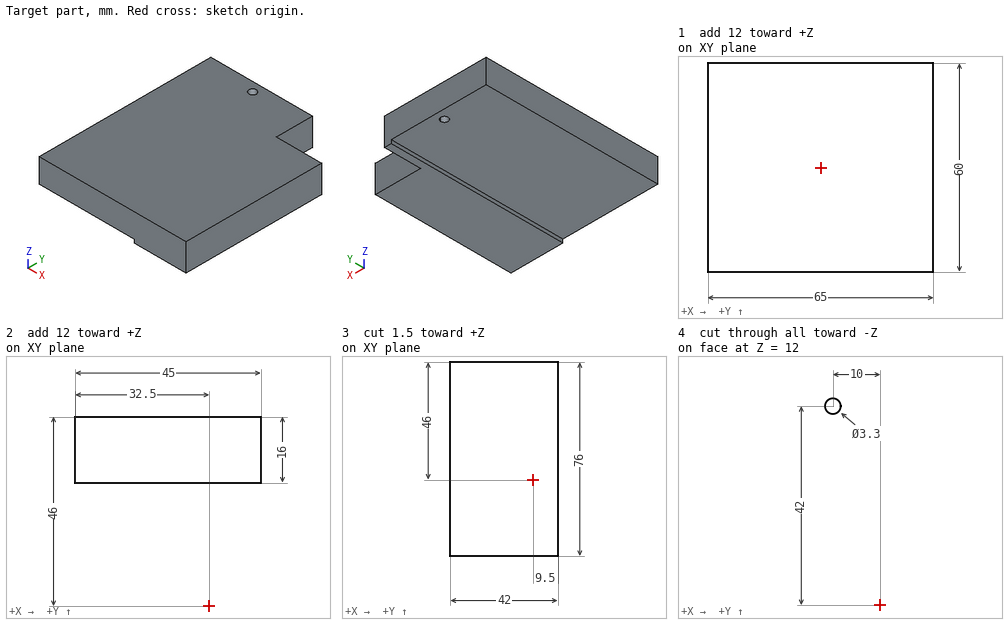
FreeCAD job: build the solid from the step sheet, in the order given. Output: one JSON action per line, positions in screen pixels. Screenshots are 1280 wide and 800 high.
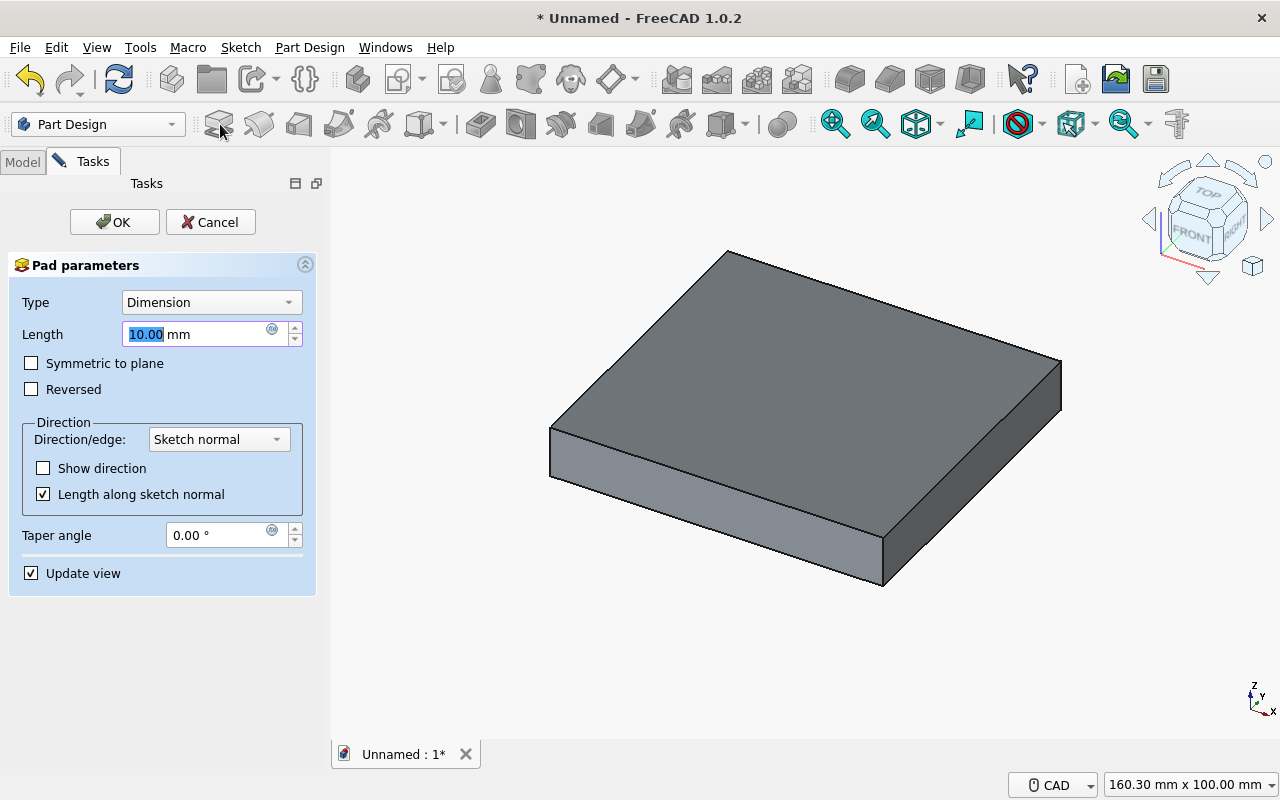
{"action": "type", "text": "12"}
{"action": "key", "text": "Tab"}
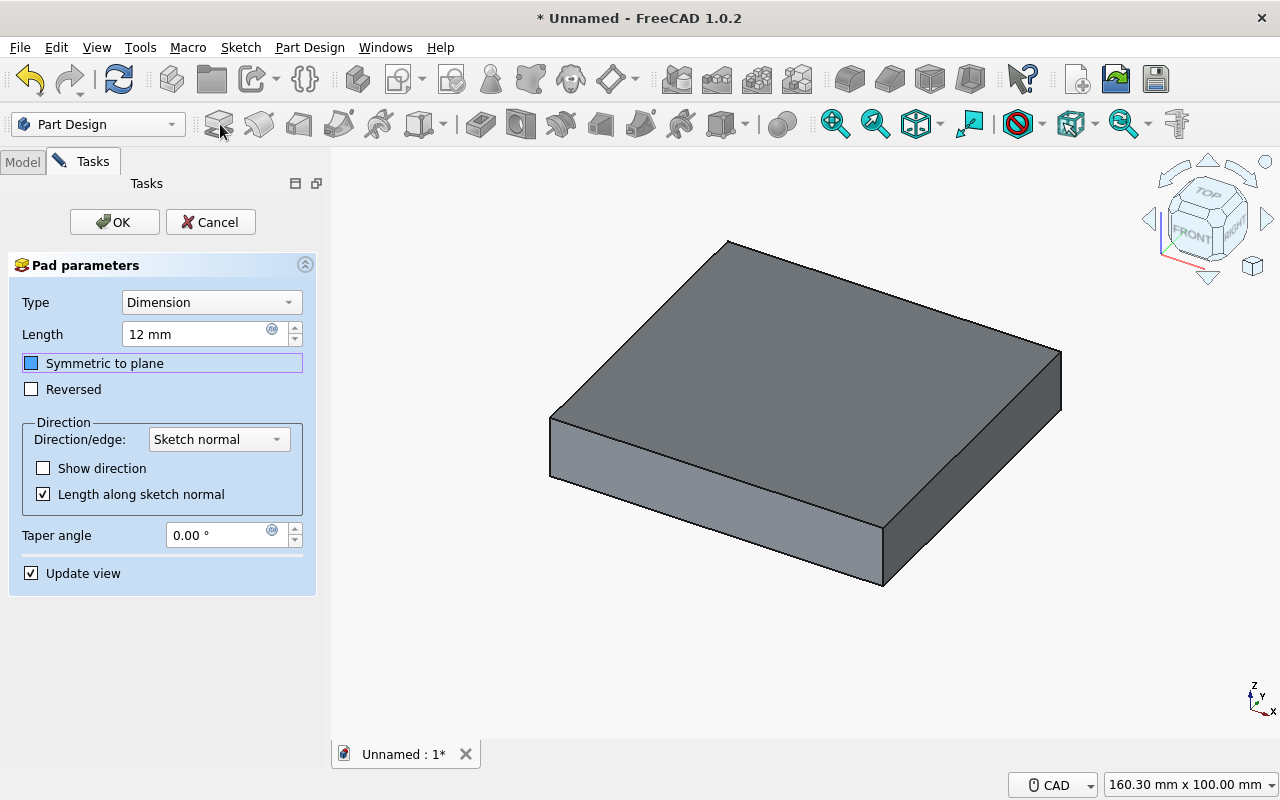
{"action": "left_click", "coordinate": [115, 222]}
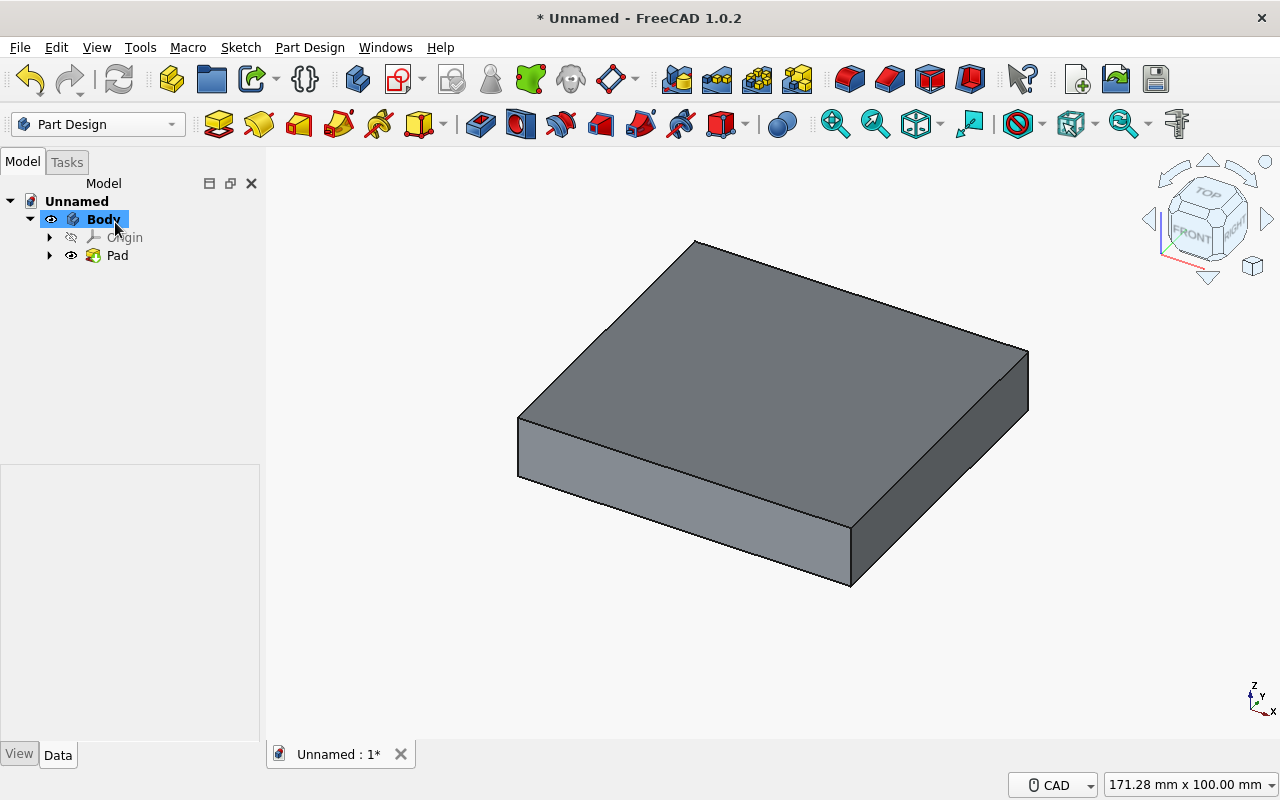
{"action": "left_click", "coordinate": [398, 80]}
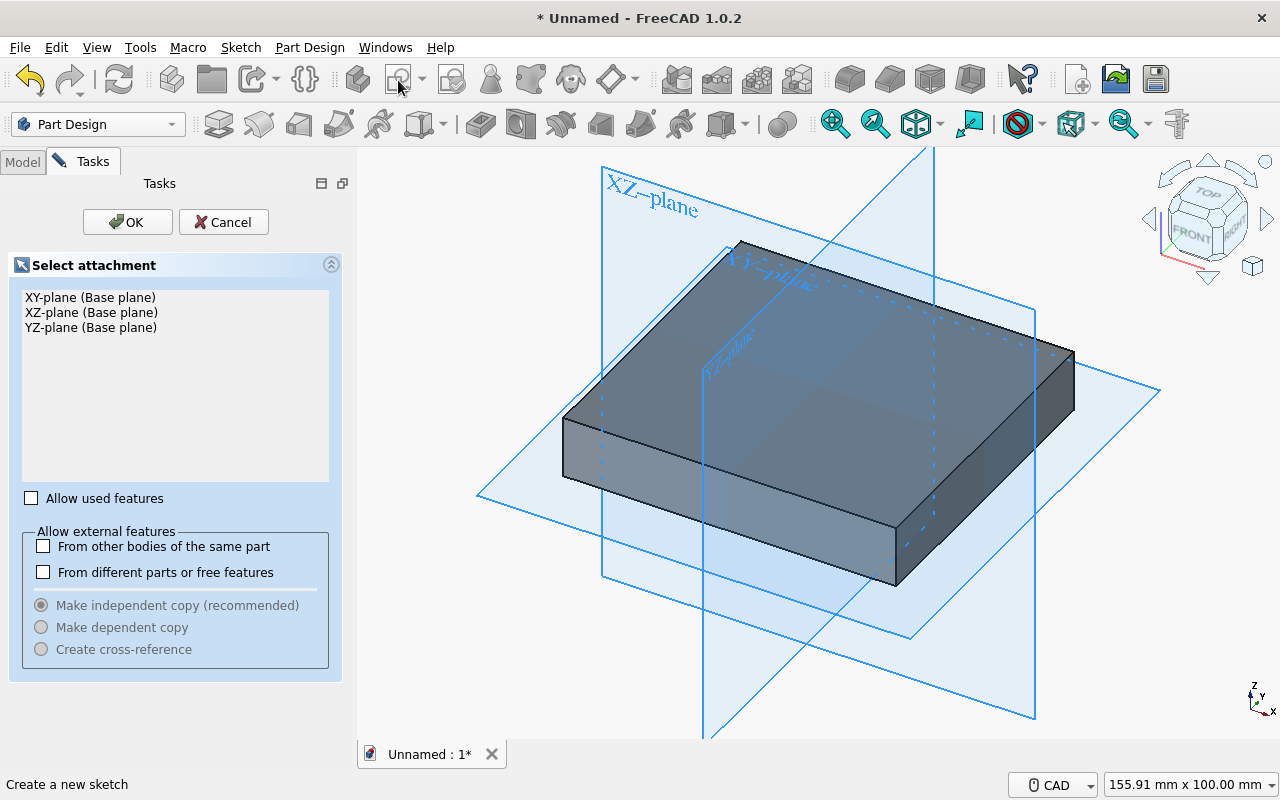
{"action": "left_click", "coordinate": [82, 298]}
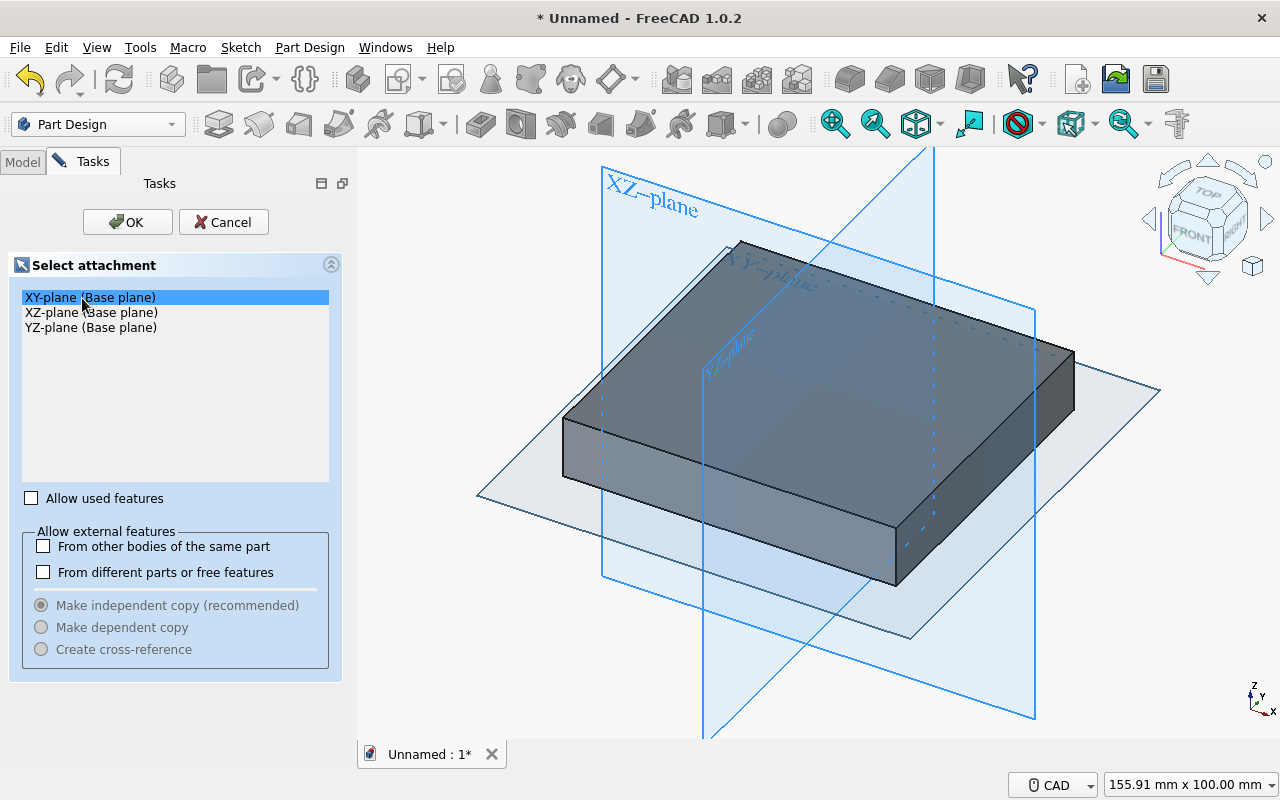
{"action": "left_click", "coordinate": [128, 222]}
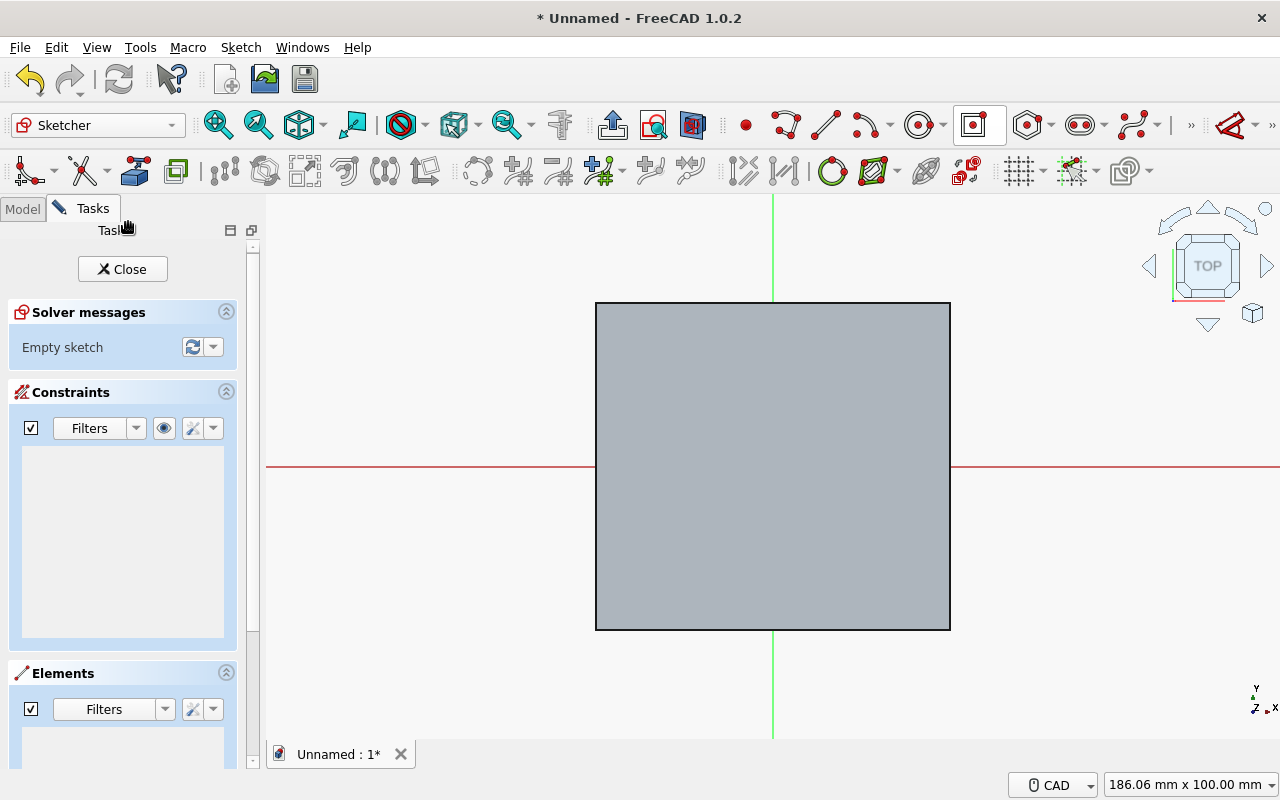
{"action": "left_click", "coordinate": [694, 126]}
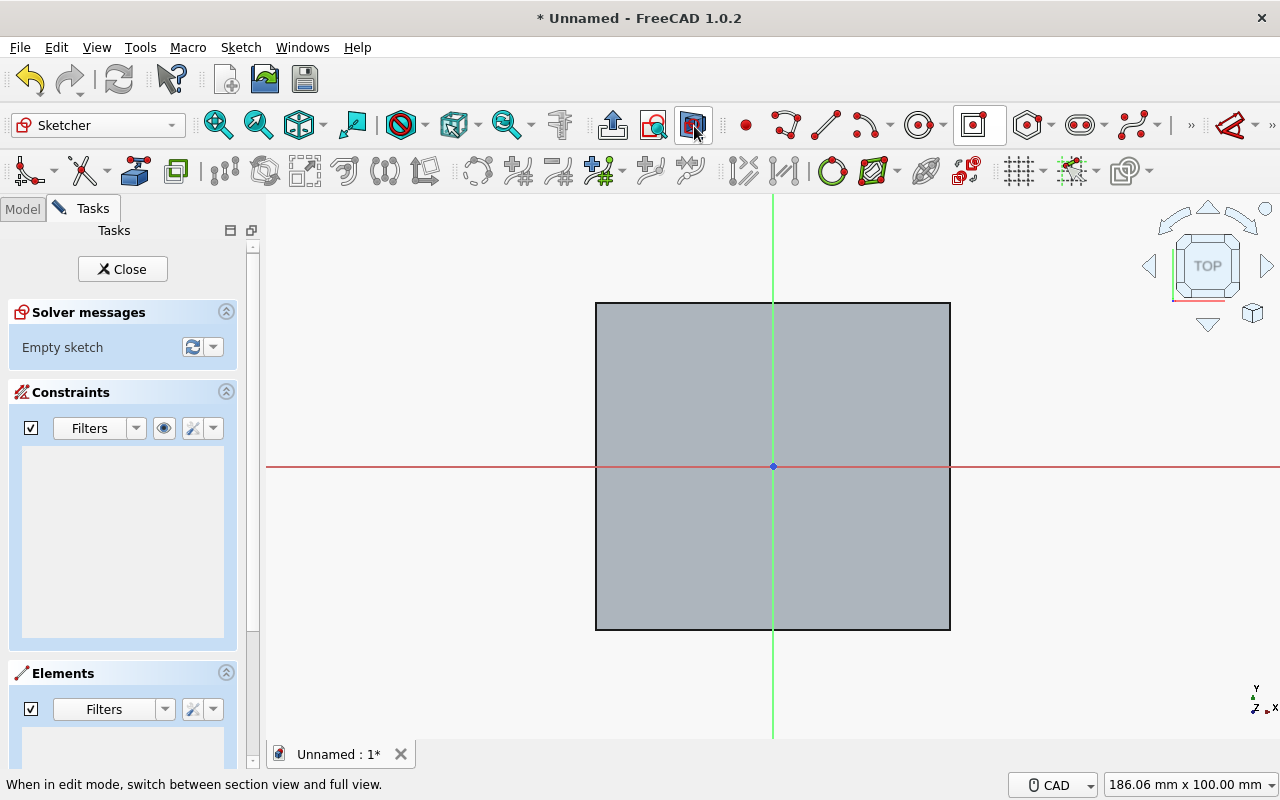
{"action": "scroll", "coordinate": [641, 711], "scroll_direction": "down", "scroll_amount": 1}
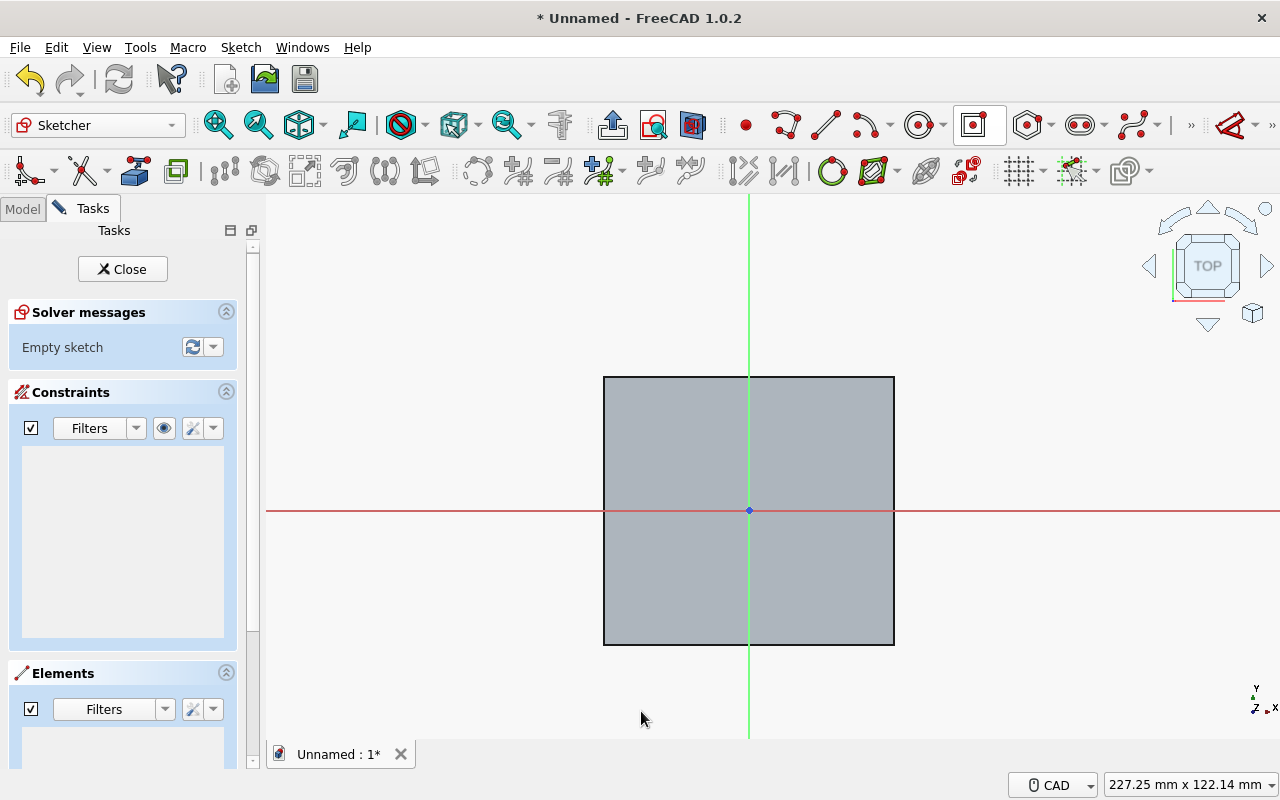
{"action": "scroll", "coordinate": [705, 338], "scroll_direction": "up", "scroll_amount": 3}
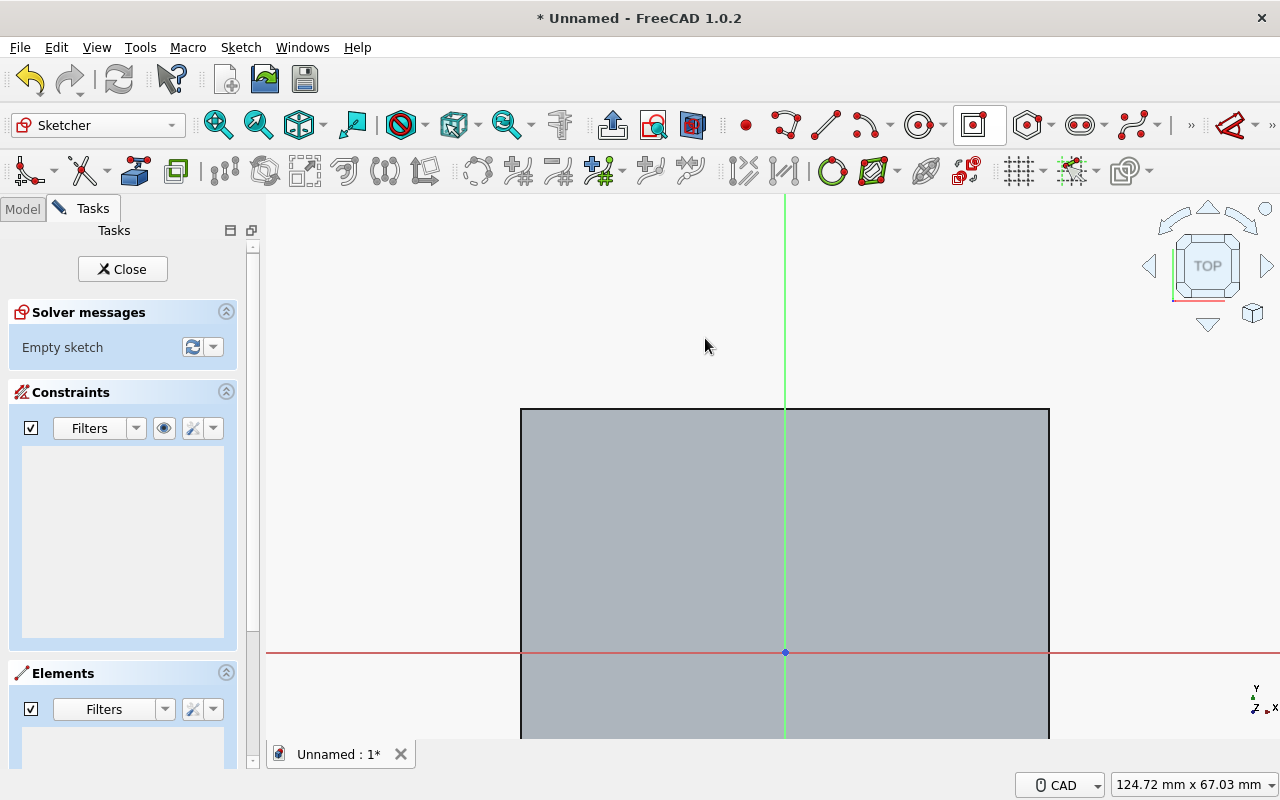
{"action": "key", "text": "g r"}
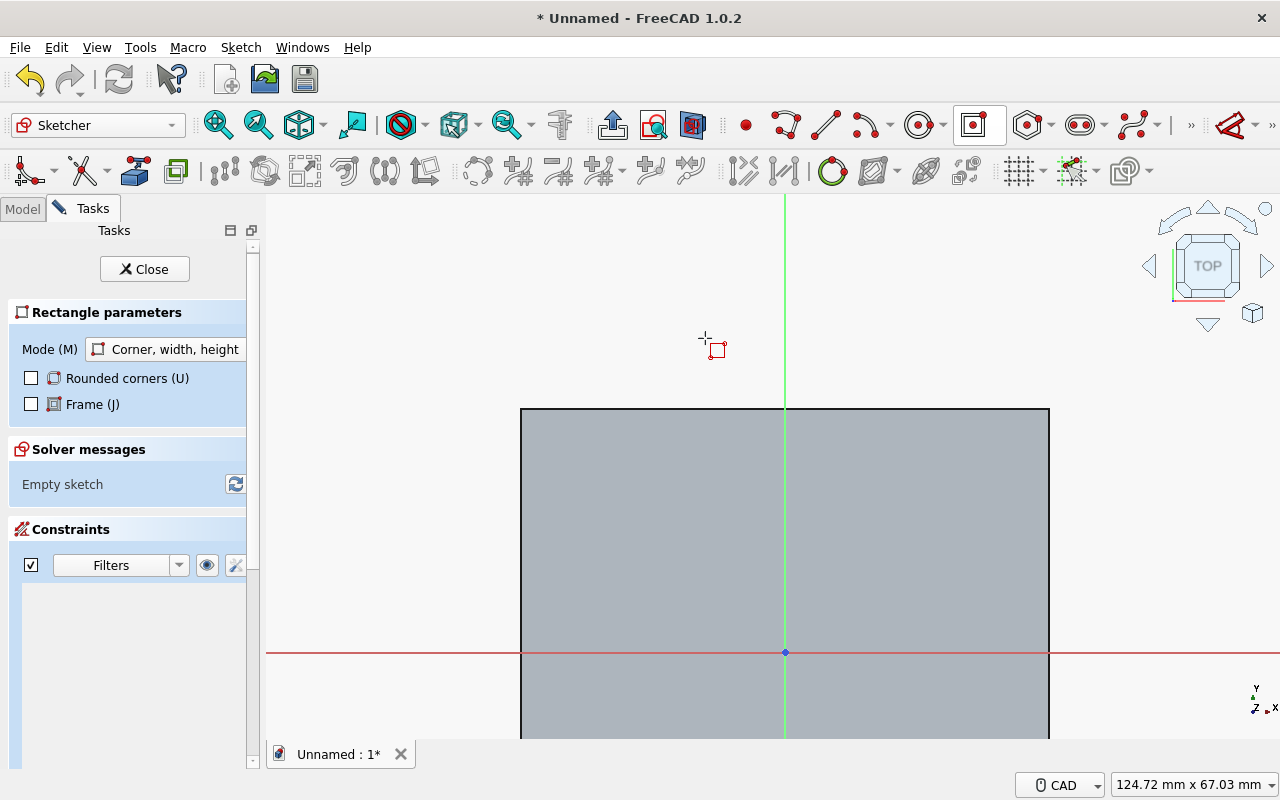
{"action": "left_click", "coordinate": [521, 279]}
{"action": "mouse_move", "coordinate": [887, 409]}